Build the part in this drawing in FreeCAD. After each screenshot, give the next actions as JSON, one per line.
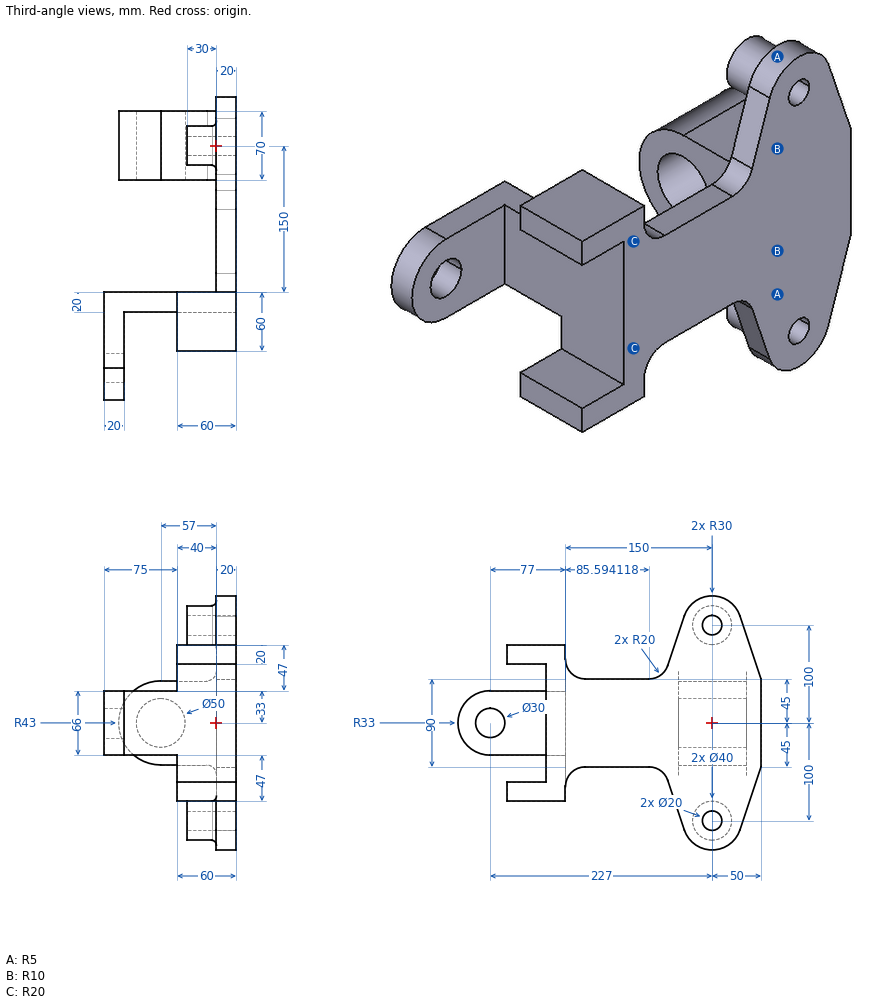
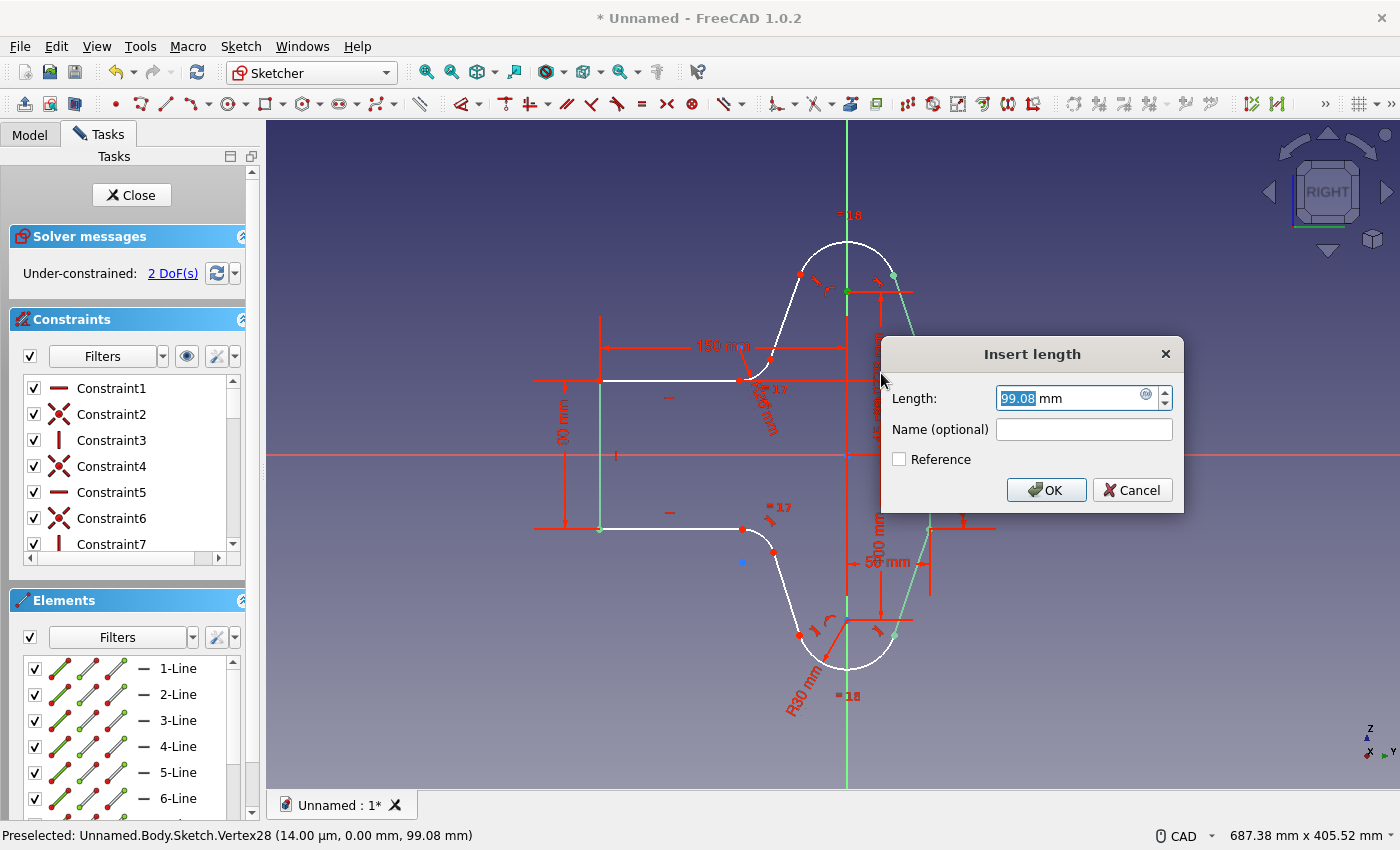
{"action": "type", "text": "100"}
{"action": "key", "text": "Return"}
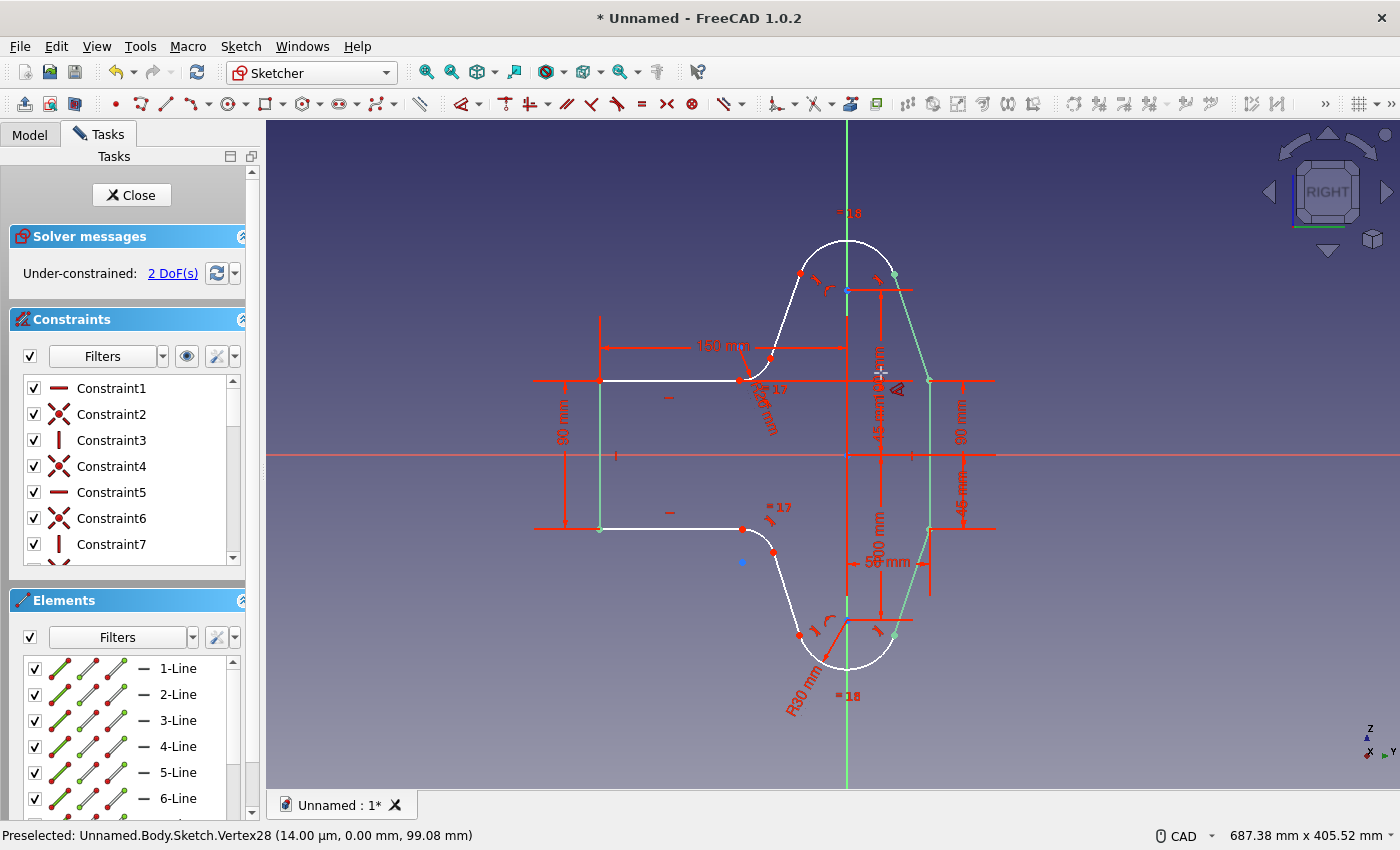
{"action": "left_click", "coordinate": [697, 381]}
{"action": "left_click", "coordinate": [637, 347]}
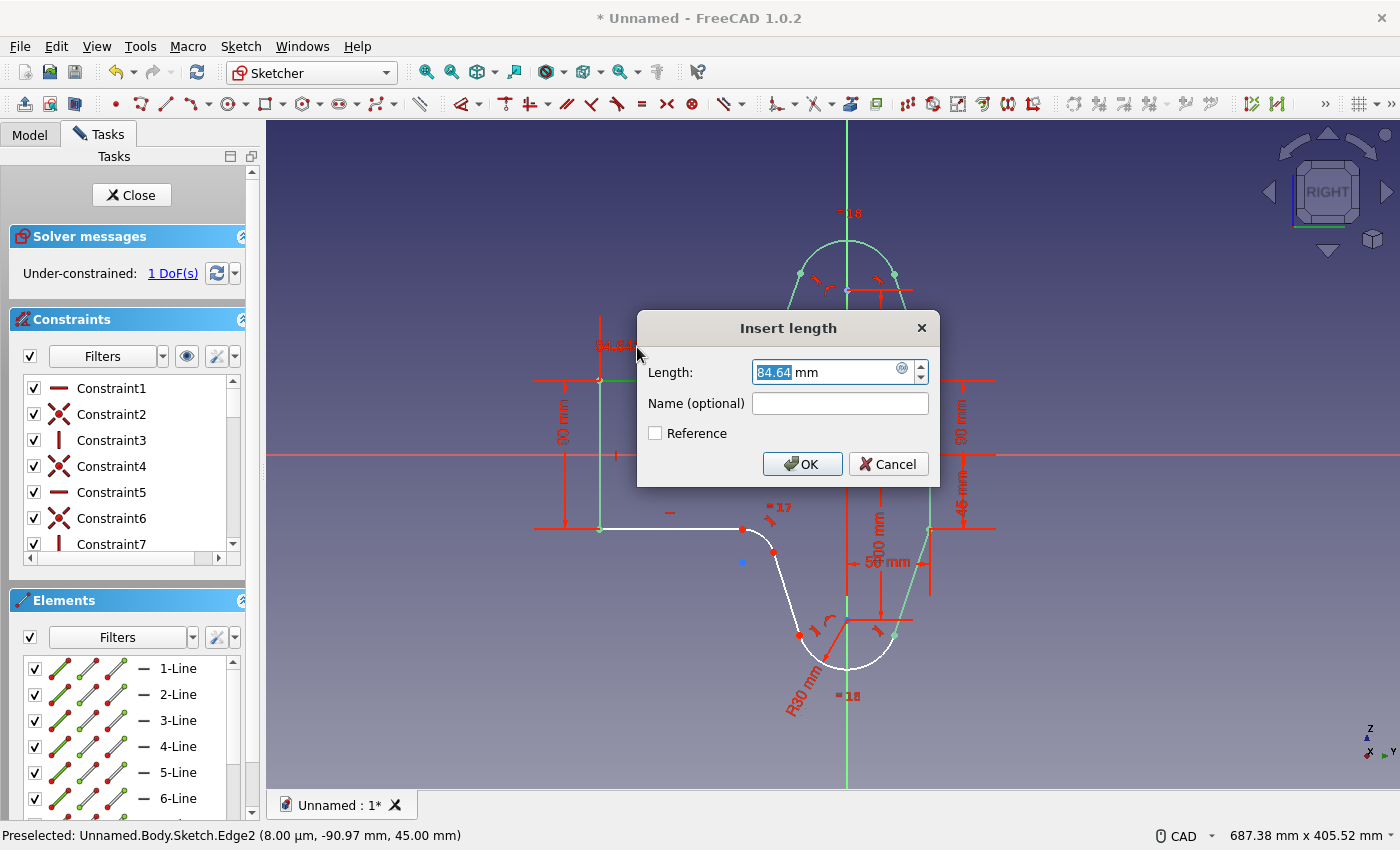
{"action": "type", "text": "85.594118"}
{"action": "key", "text": "Return"}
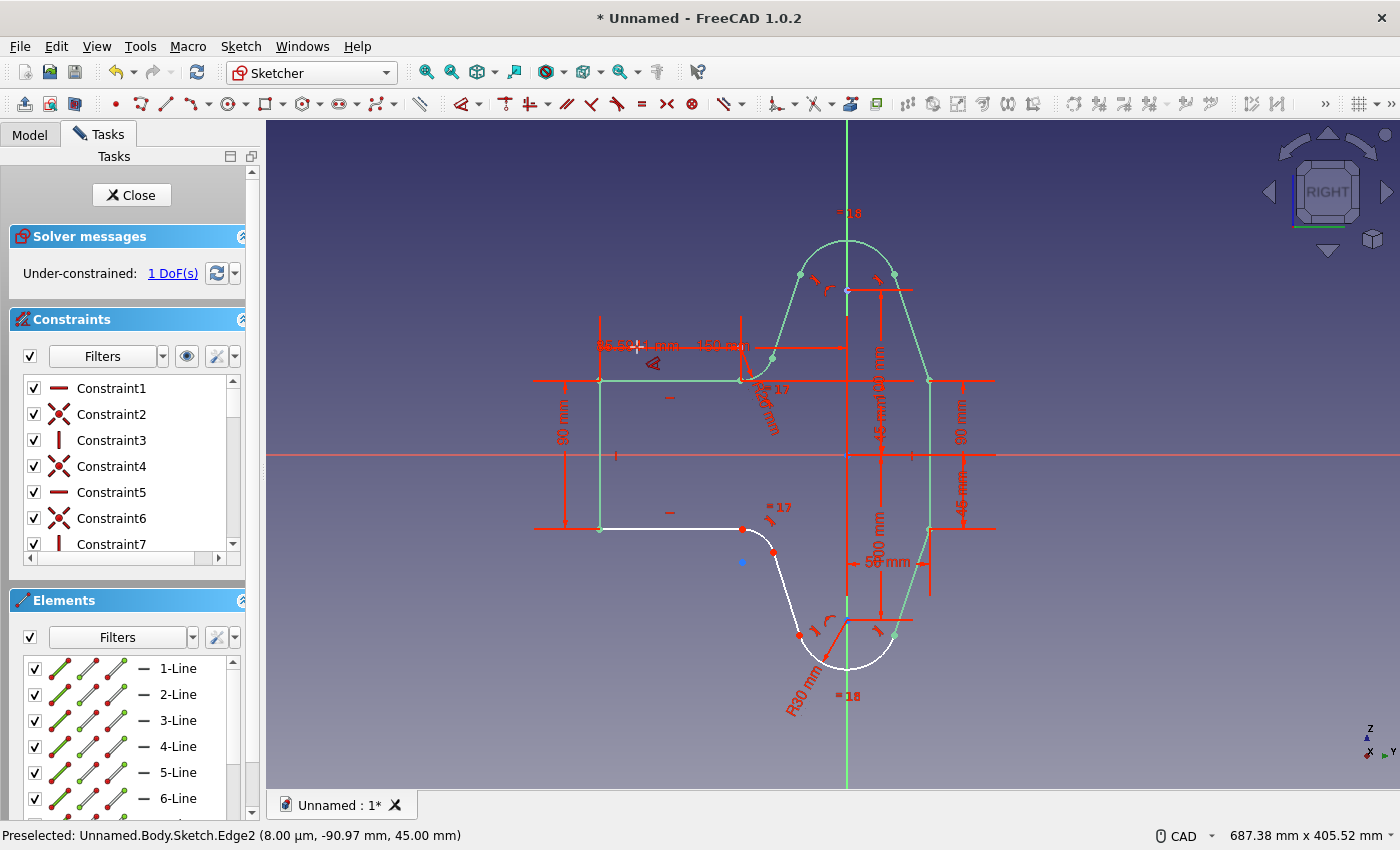
{"action": "left_click", "coordinate": [642, 529]}
{"action": "left_click", "coordinate": [671, 563]}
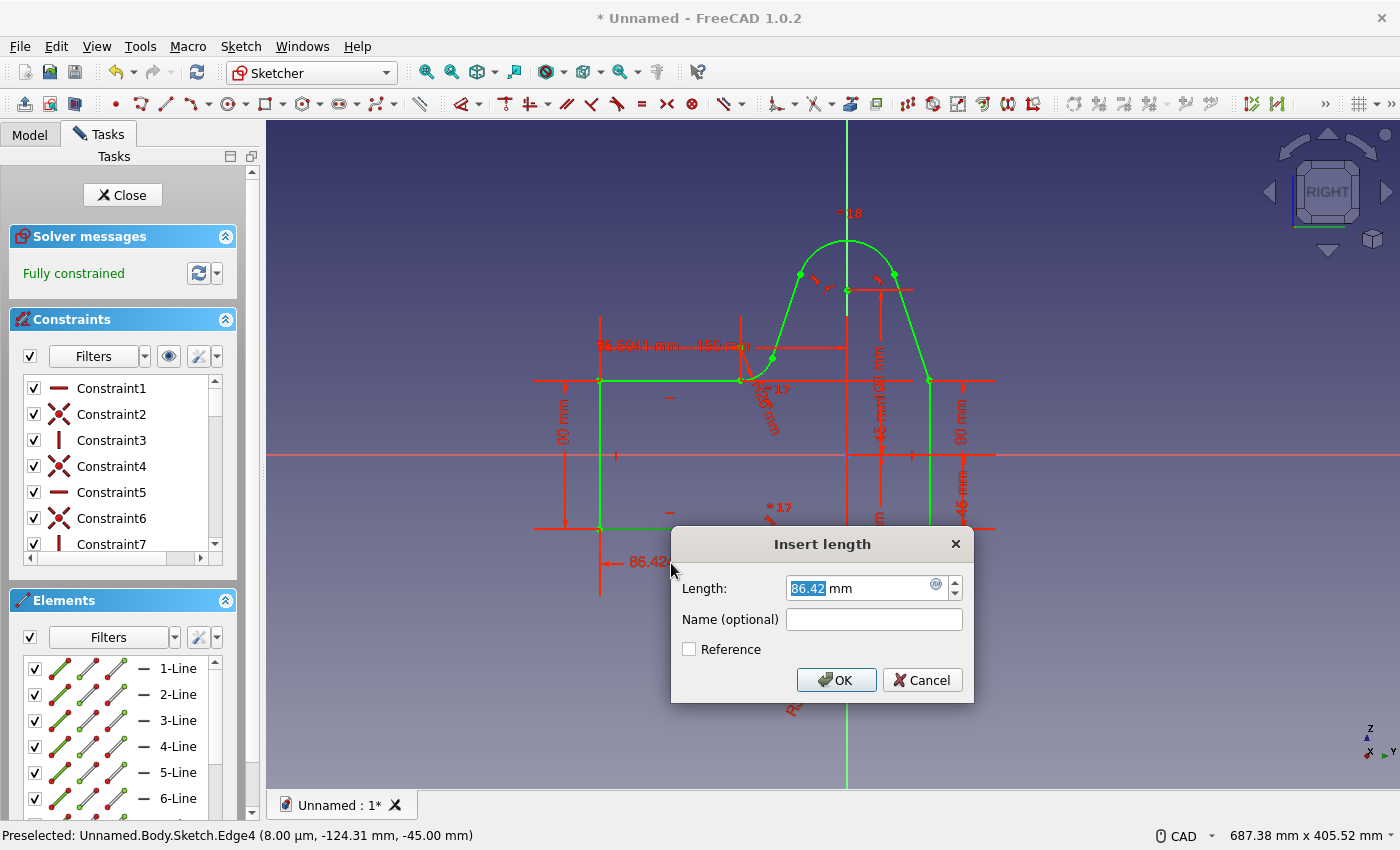
{"action": "type", "text": "85.594118"}
{"action": "key", "text": "Return"}
{"action": "key", "text": "Escape"}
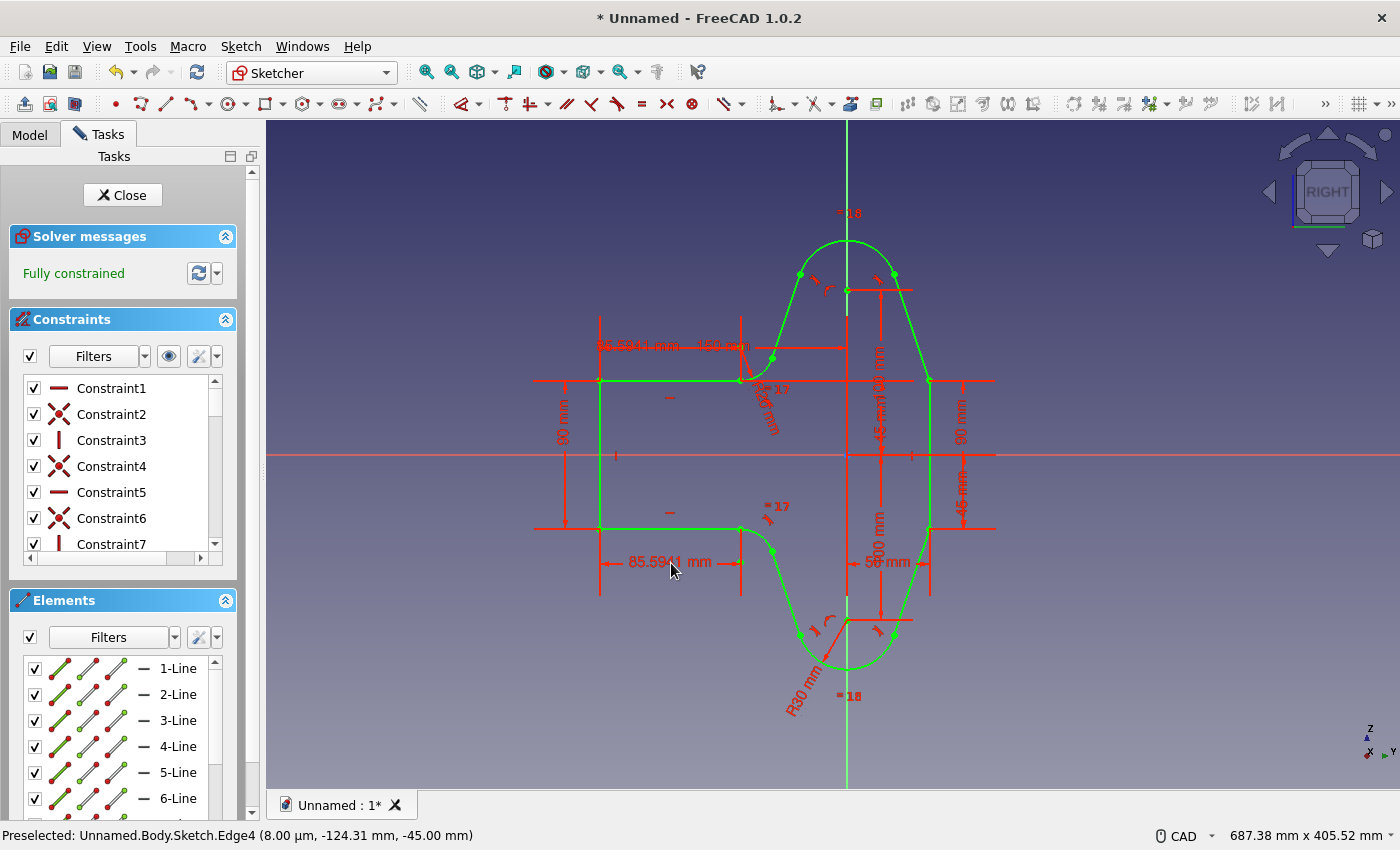
{"action": "left_click", "coordinate": [123, 195]}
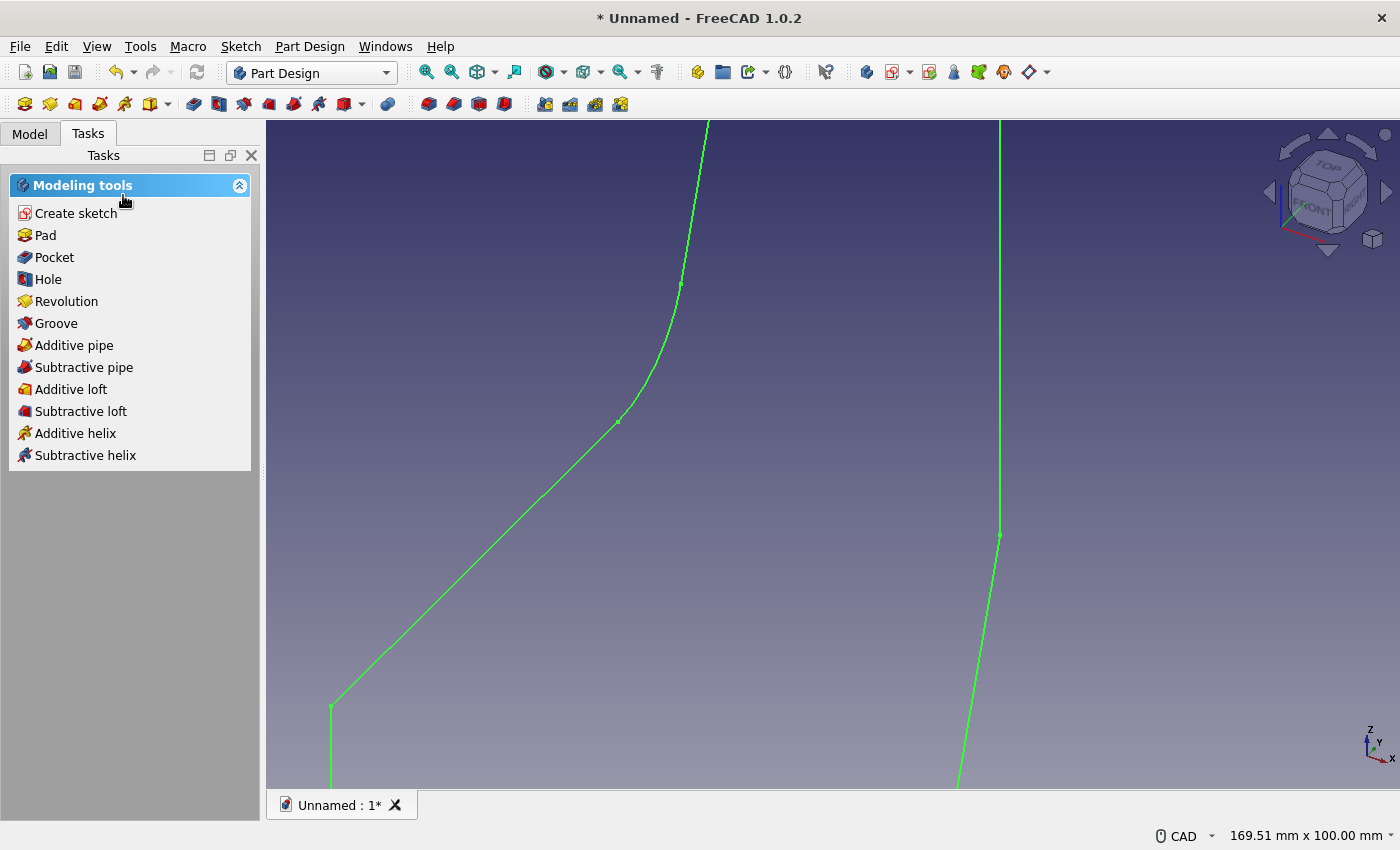
{"action": "left_click", "coordinate": [25, 104]}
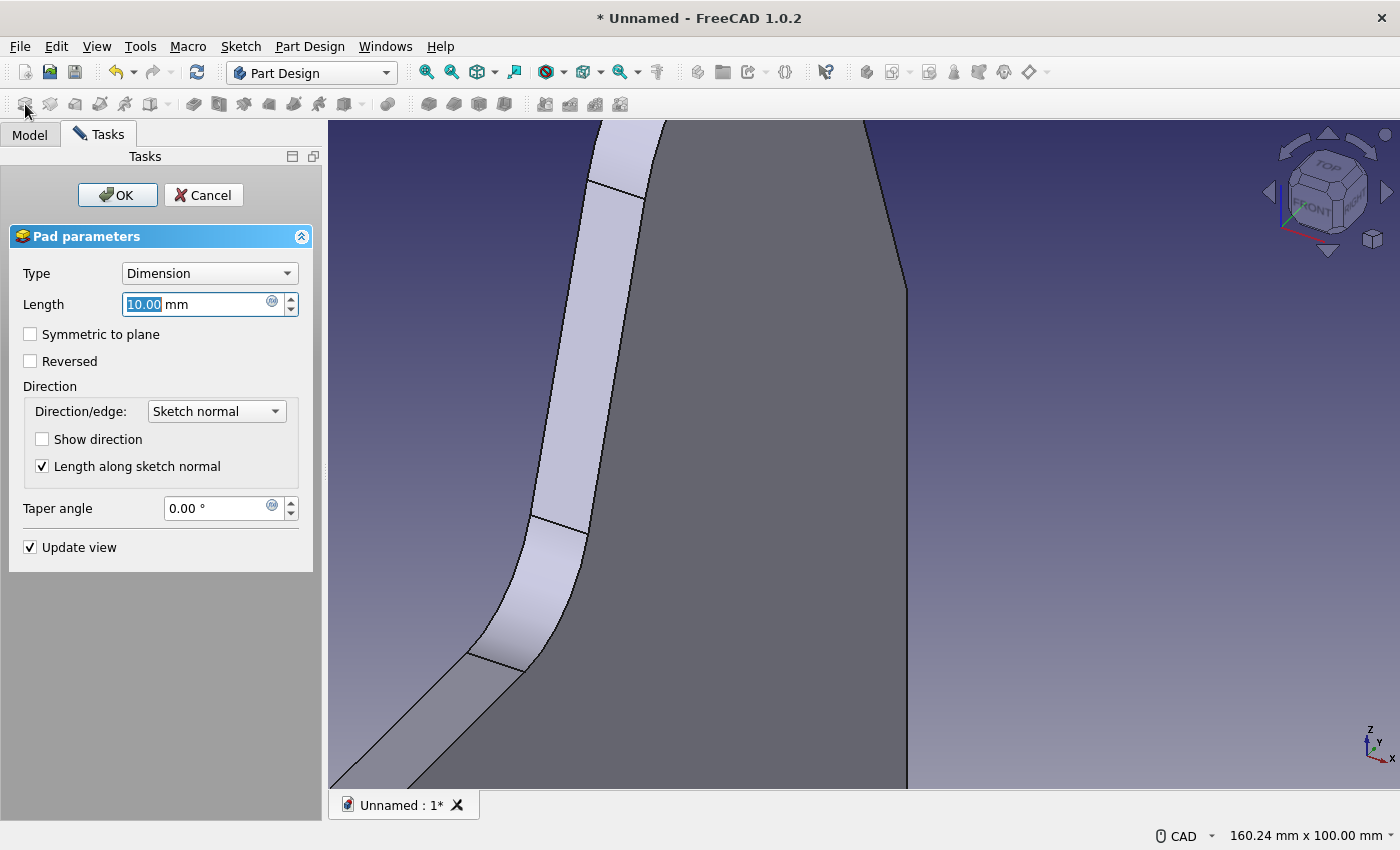
{"action": "type", "text": "20"}
{"action": "key", "text": "Tab"}